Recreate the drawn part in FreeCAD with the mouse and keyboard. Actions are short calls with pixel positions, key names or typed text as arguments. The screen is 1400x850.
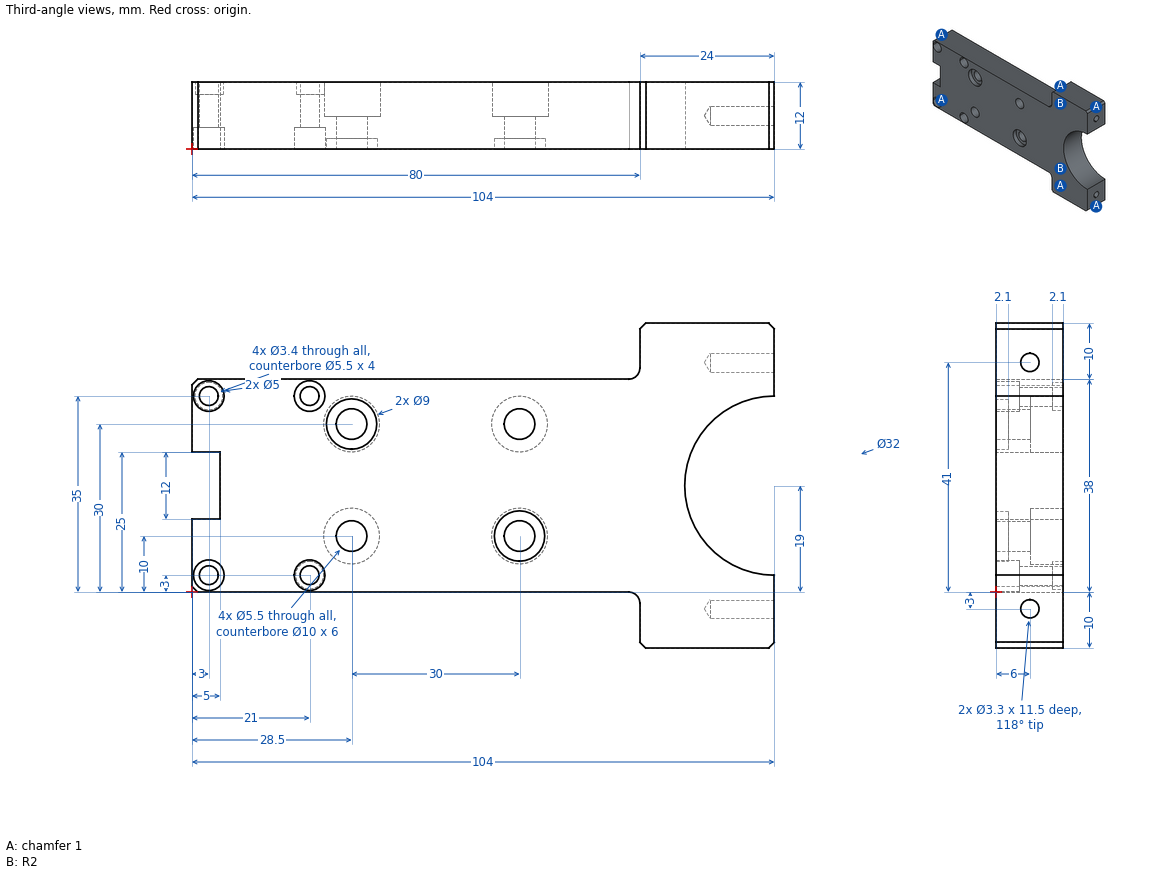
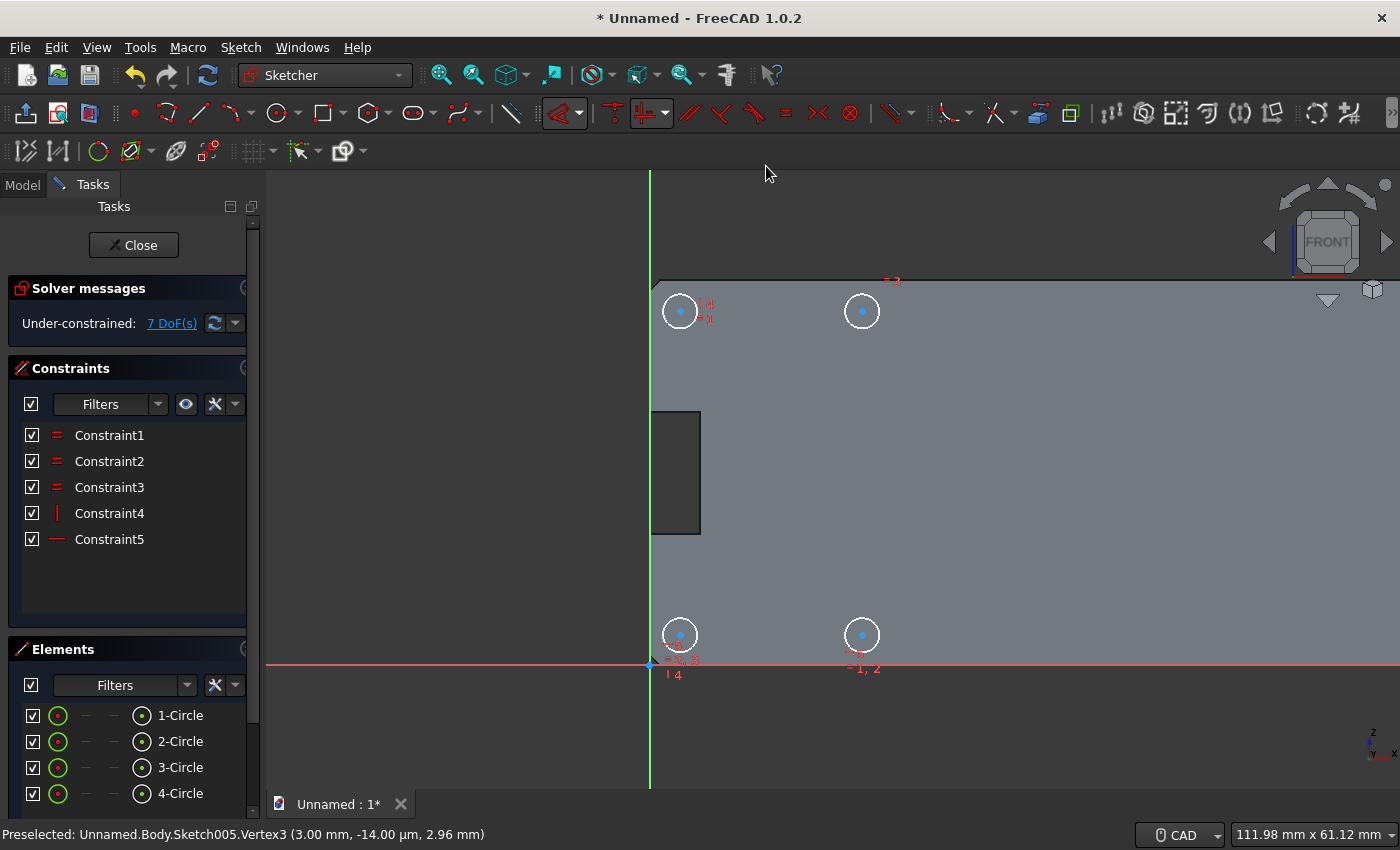
click(862, 635)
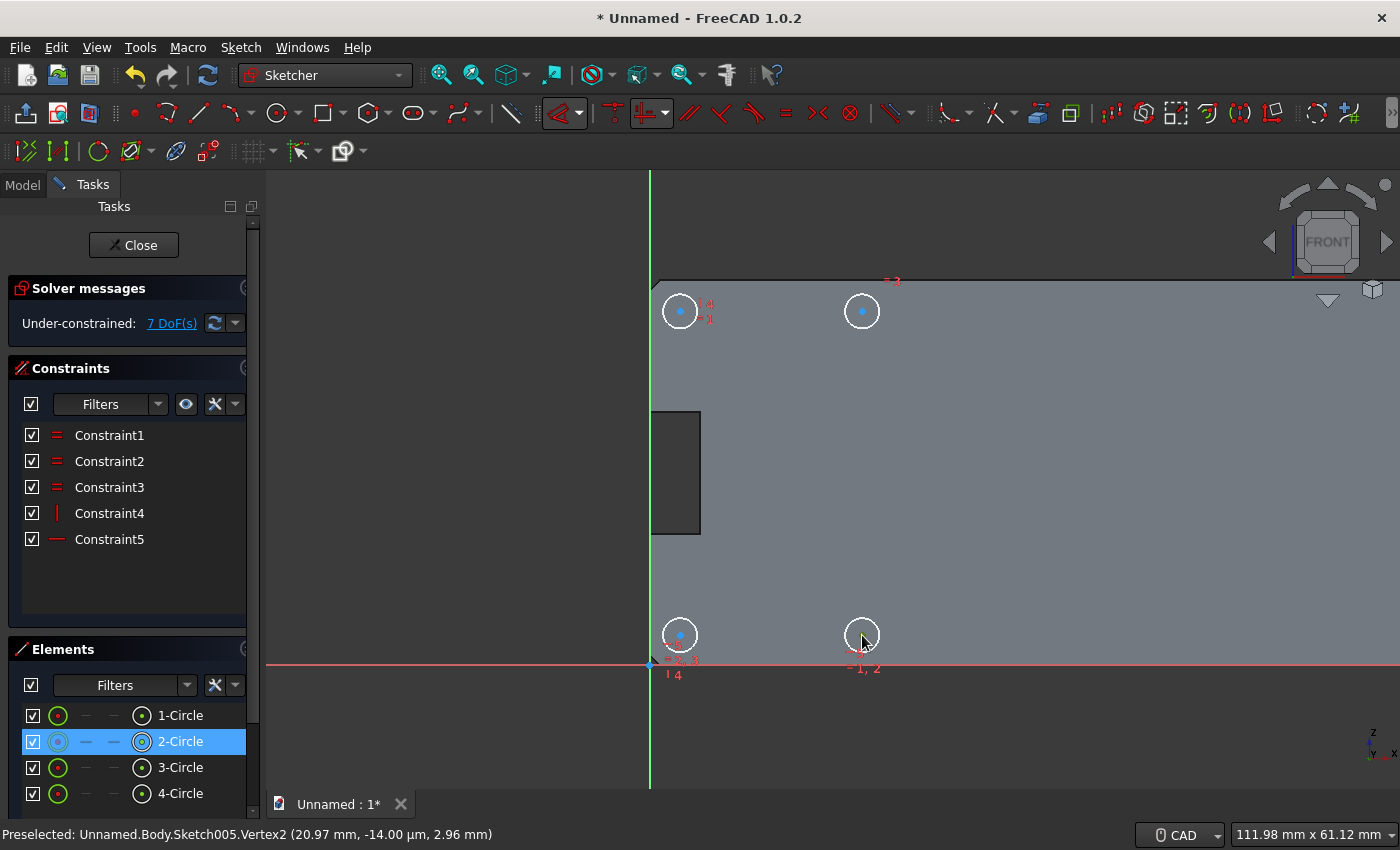
click(862, 311)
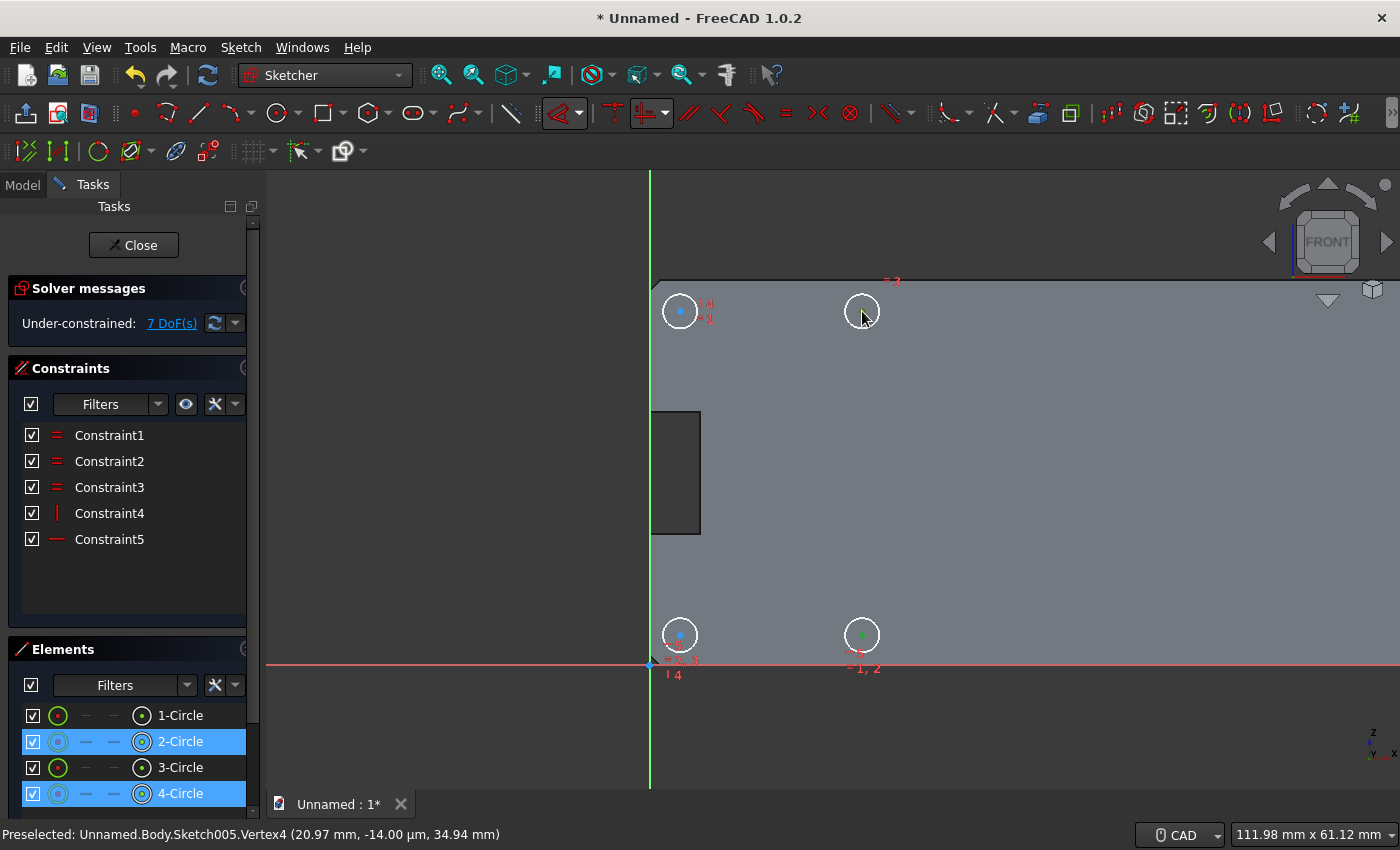
click(668, 114)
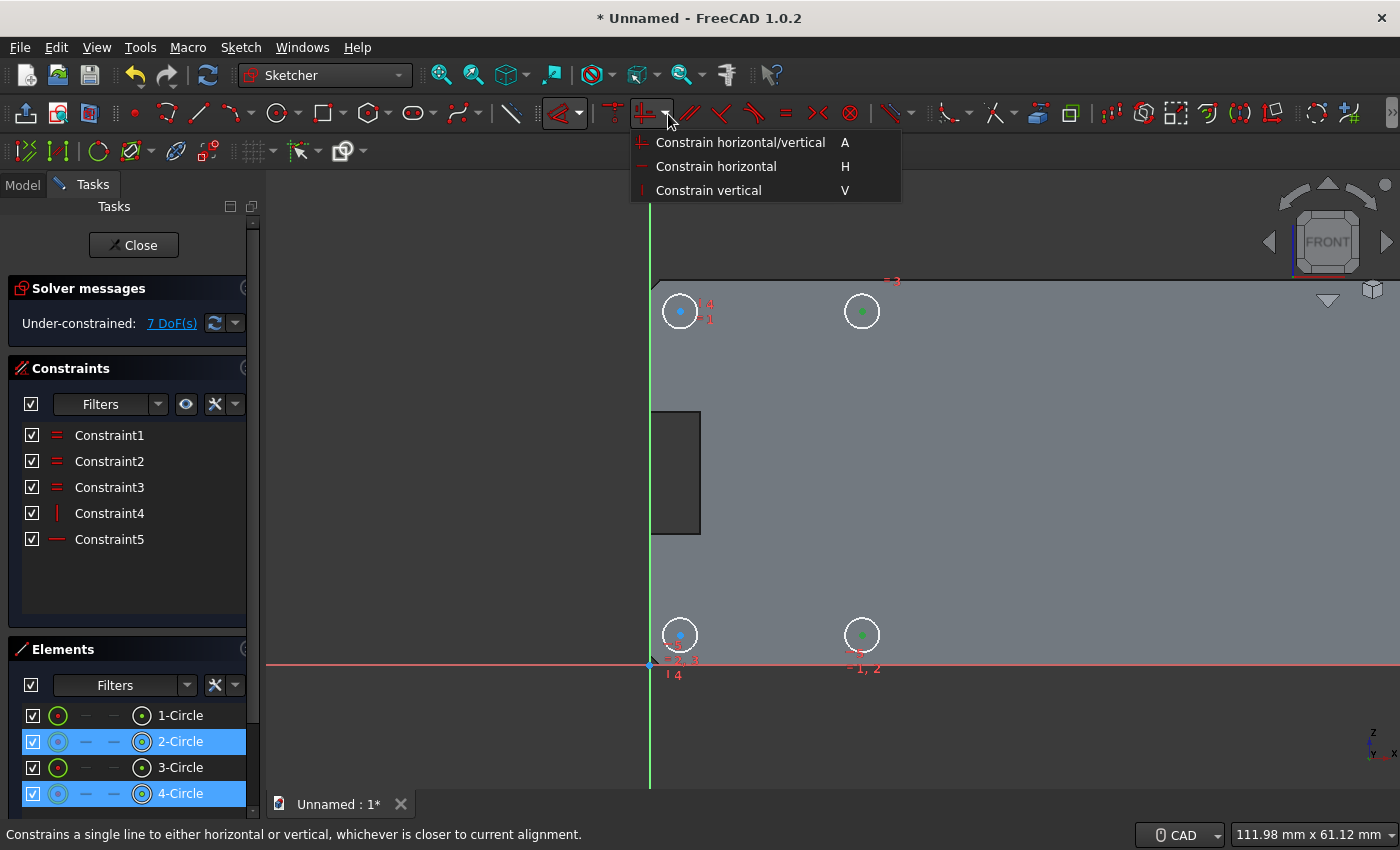
click(766, 190)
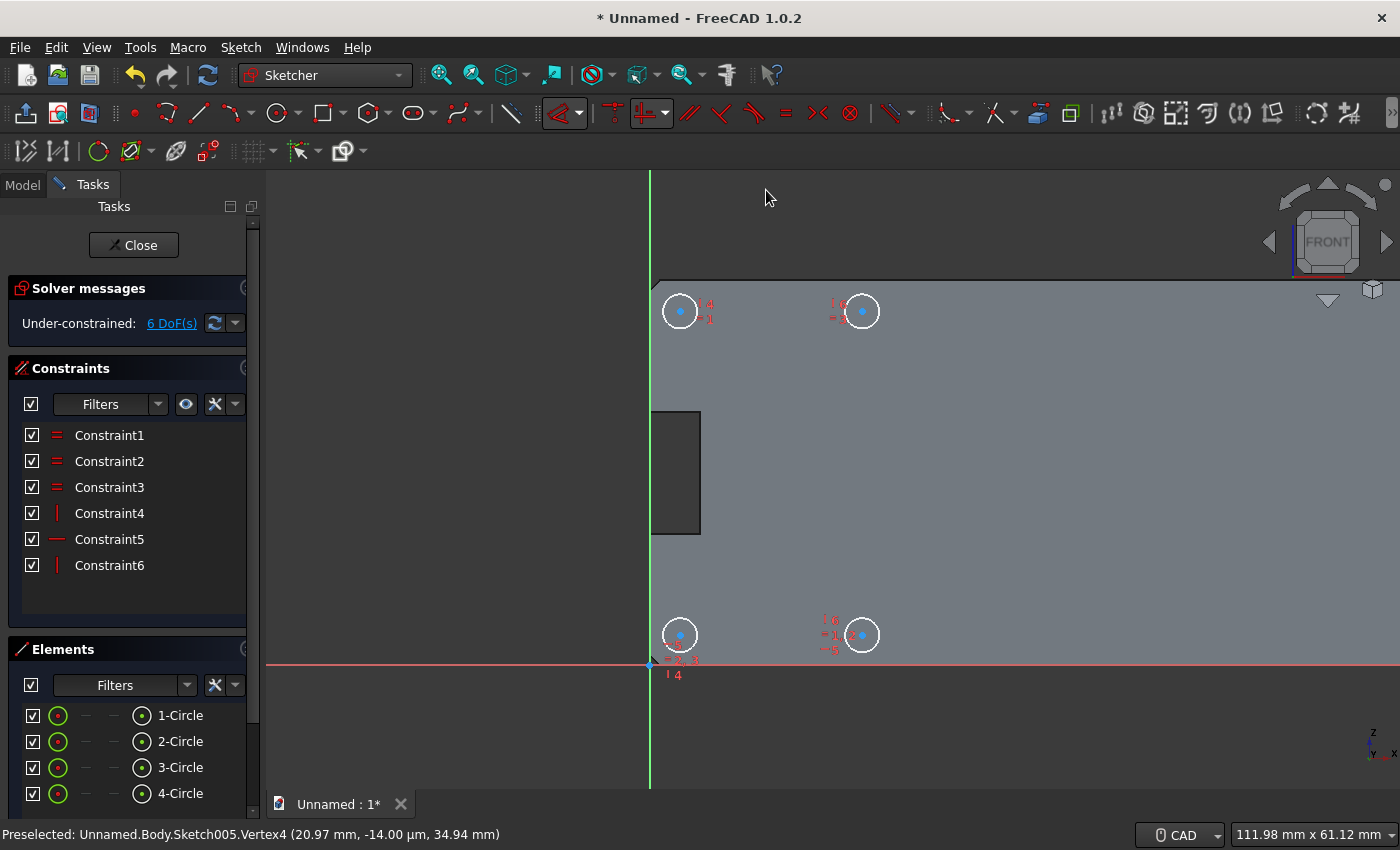
click(680, 311)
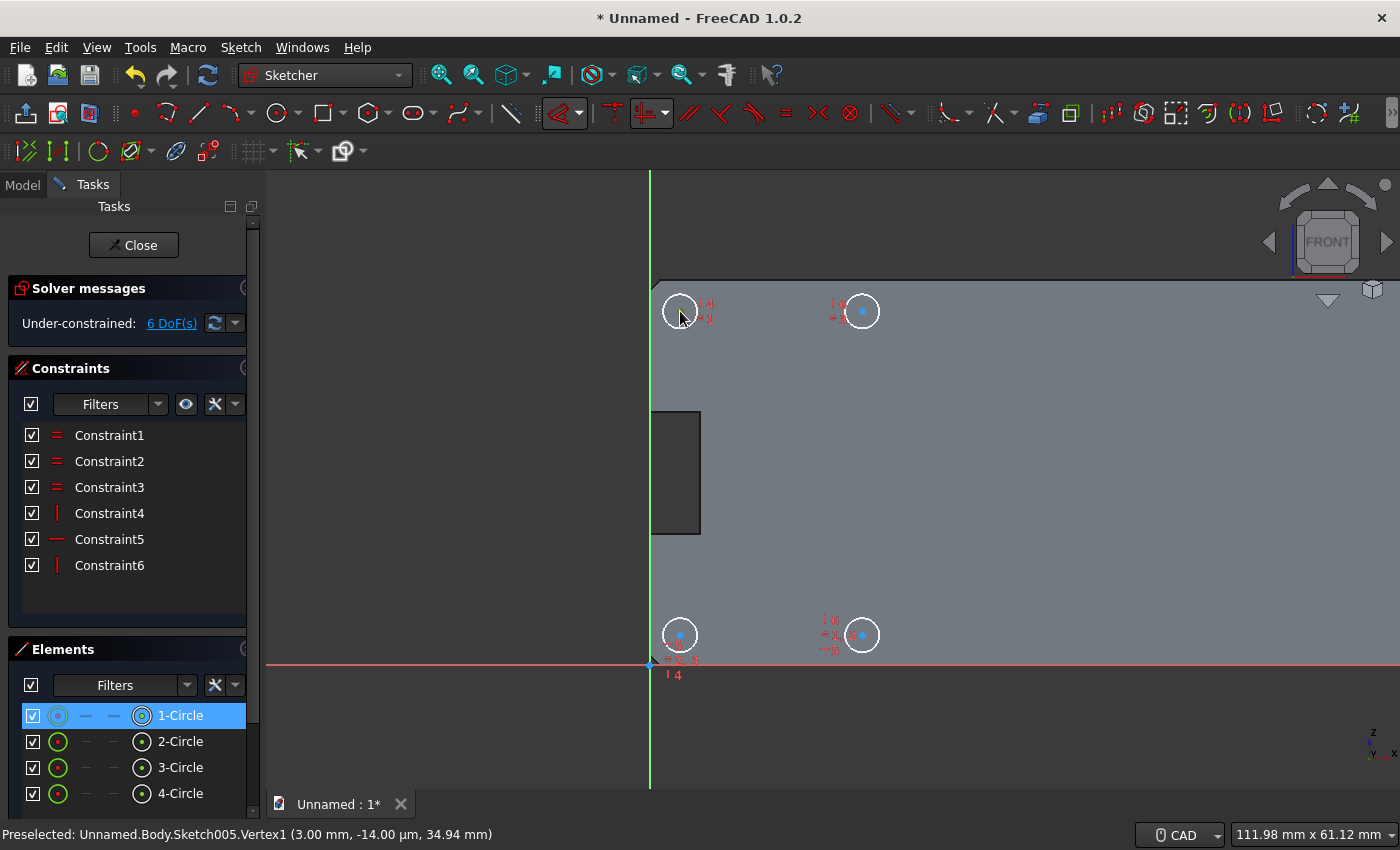
click(862, 311)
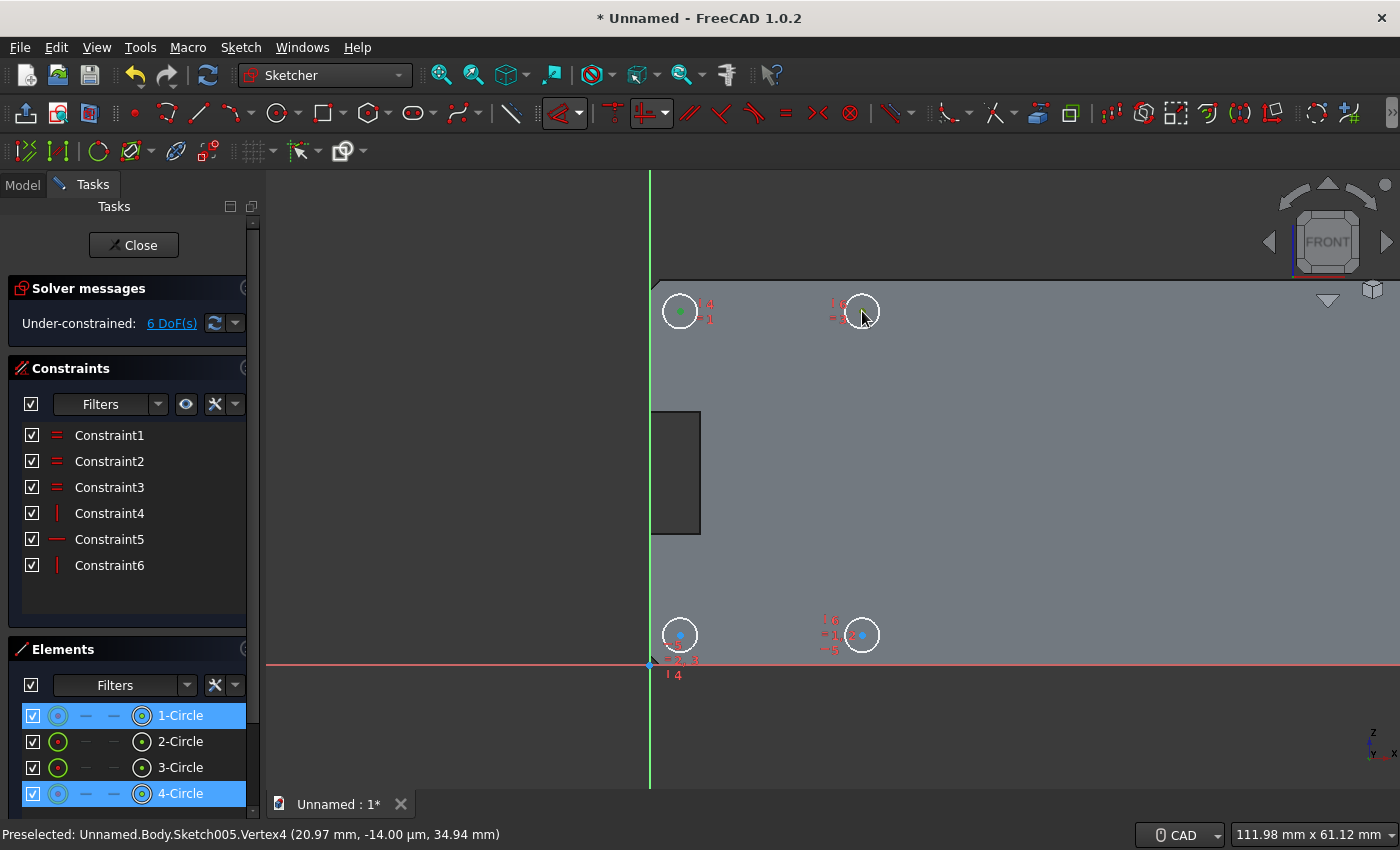
click(668, 114)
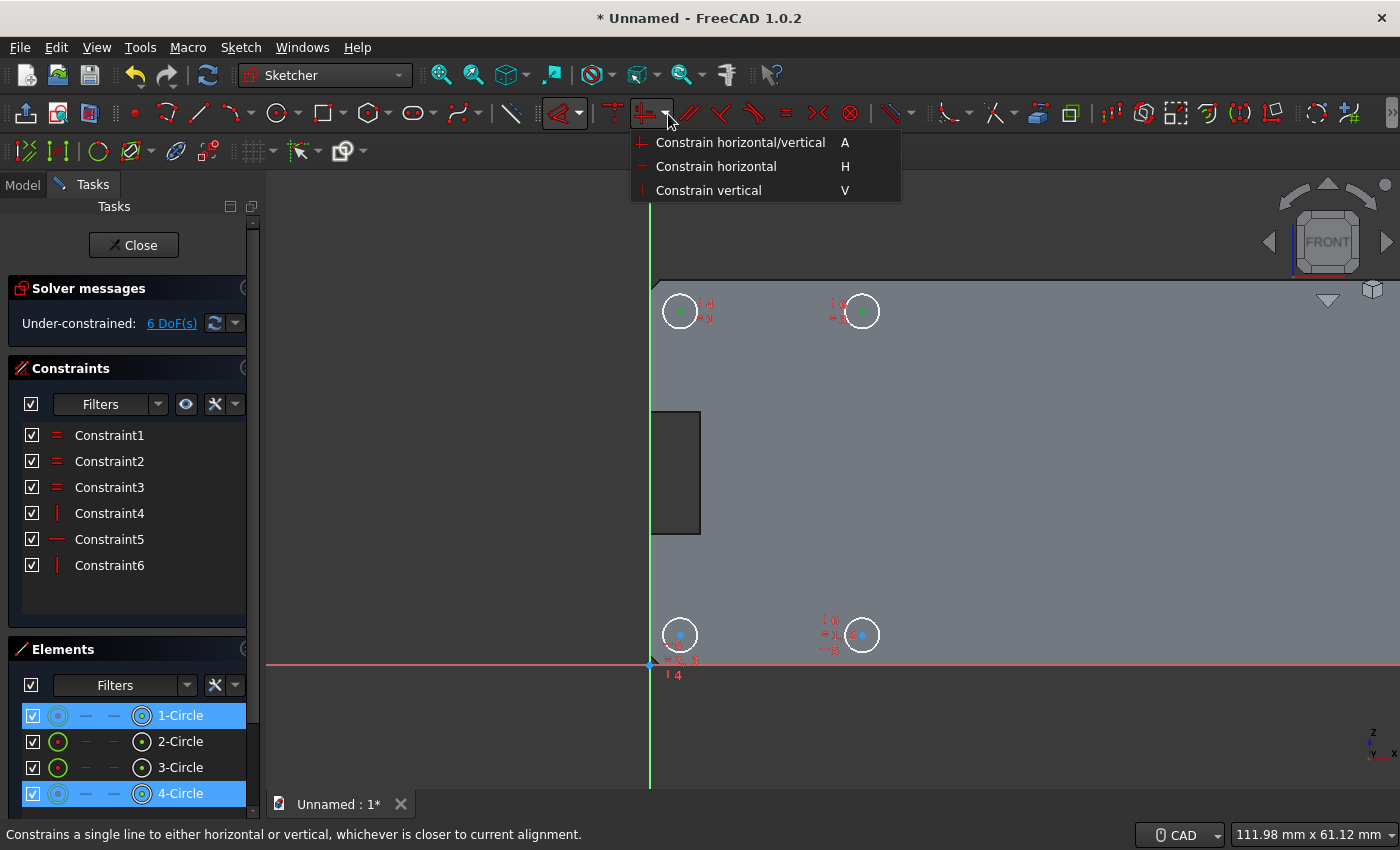
click(766, 166)